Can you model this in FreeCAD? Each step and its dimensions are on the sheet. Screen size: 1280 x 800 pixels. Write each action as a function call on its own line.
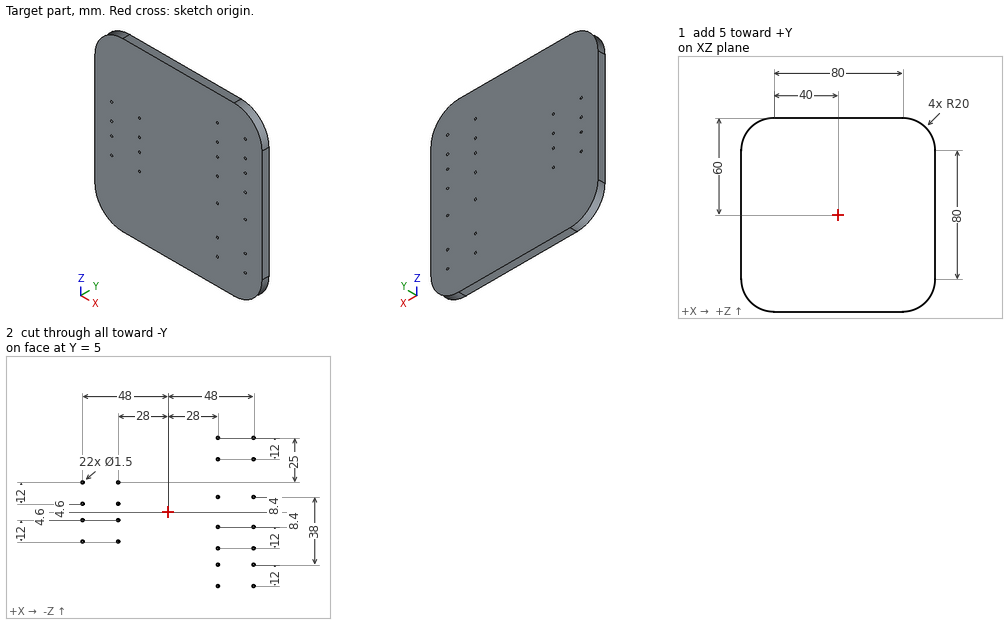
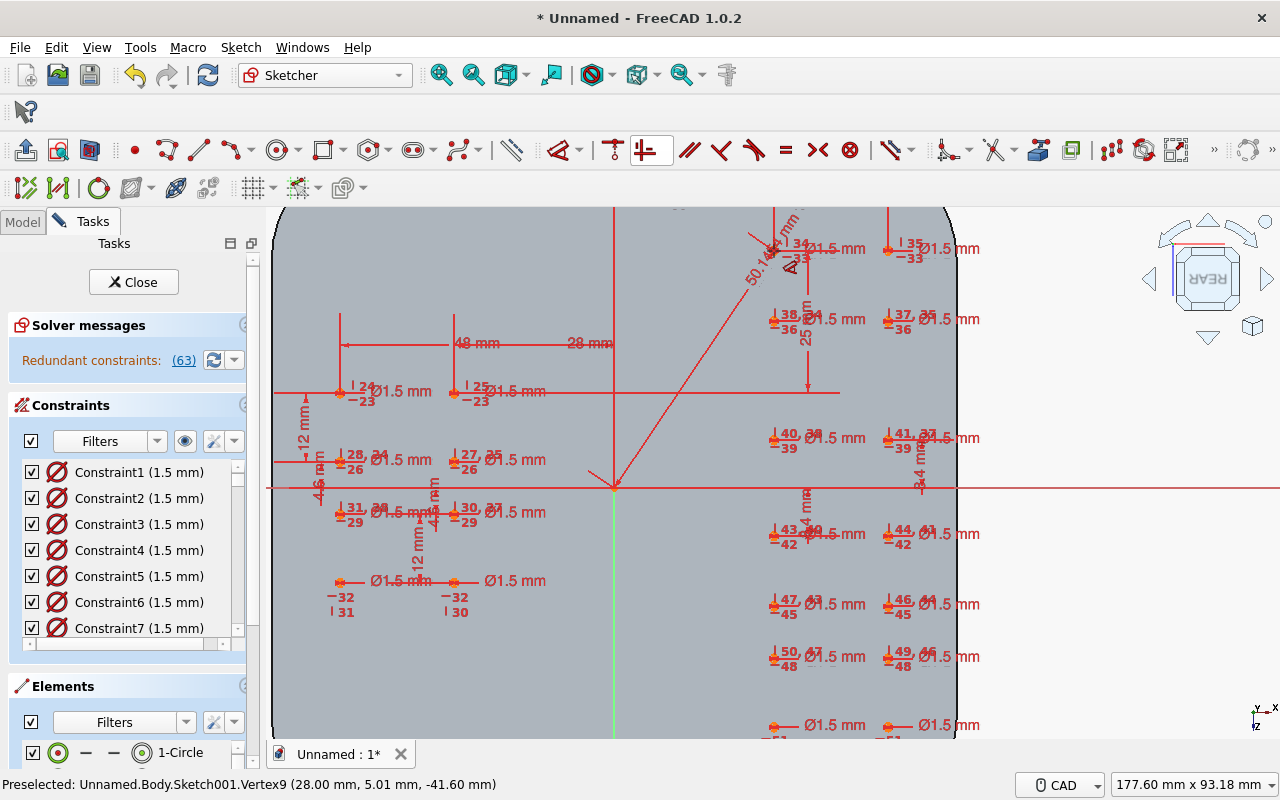
click(774, 321)
click(808, 286)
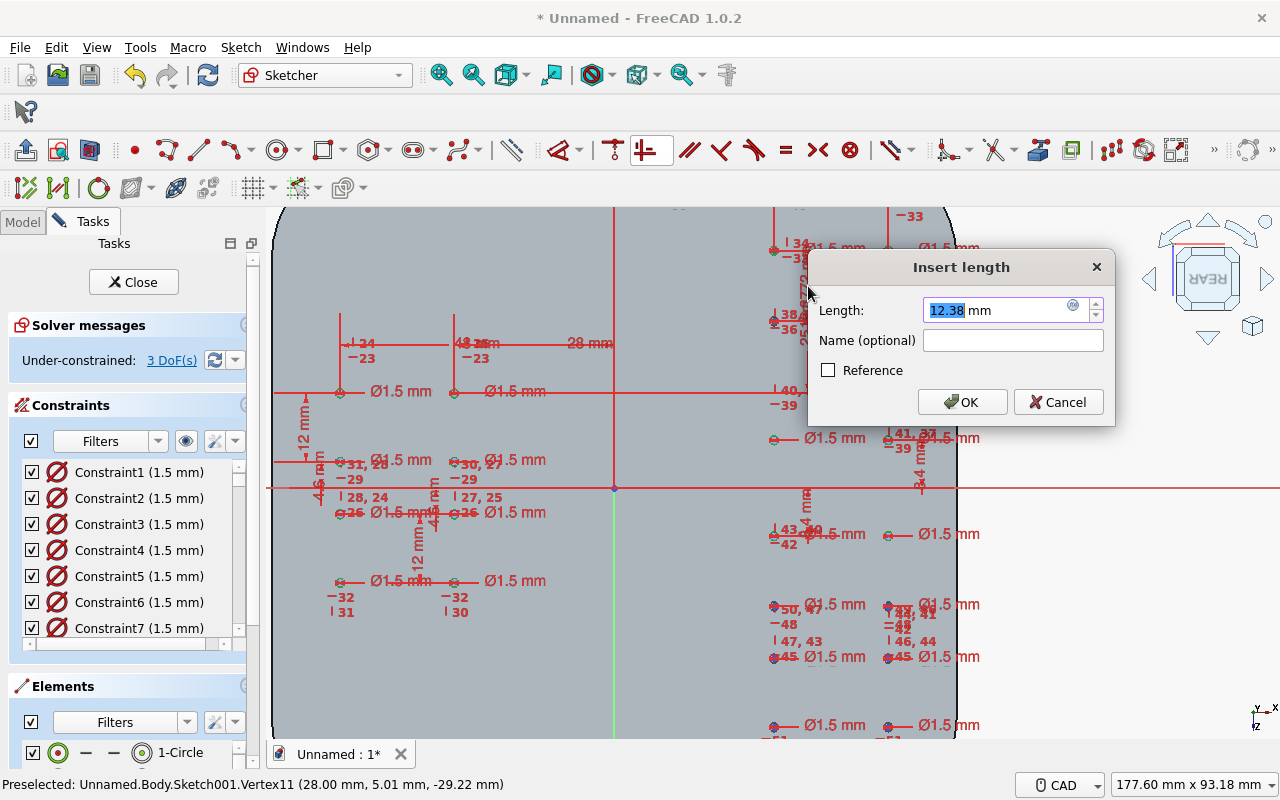
text(12)
key(Return)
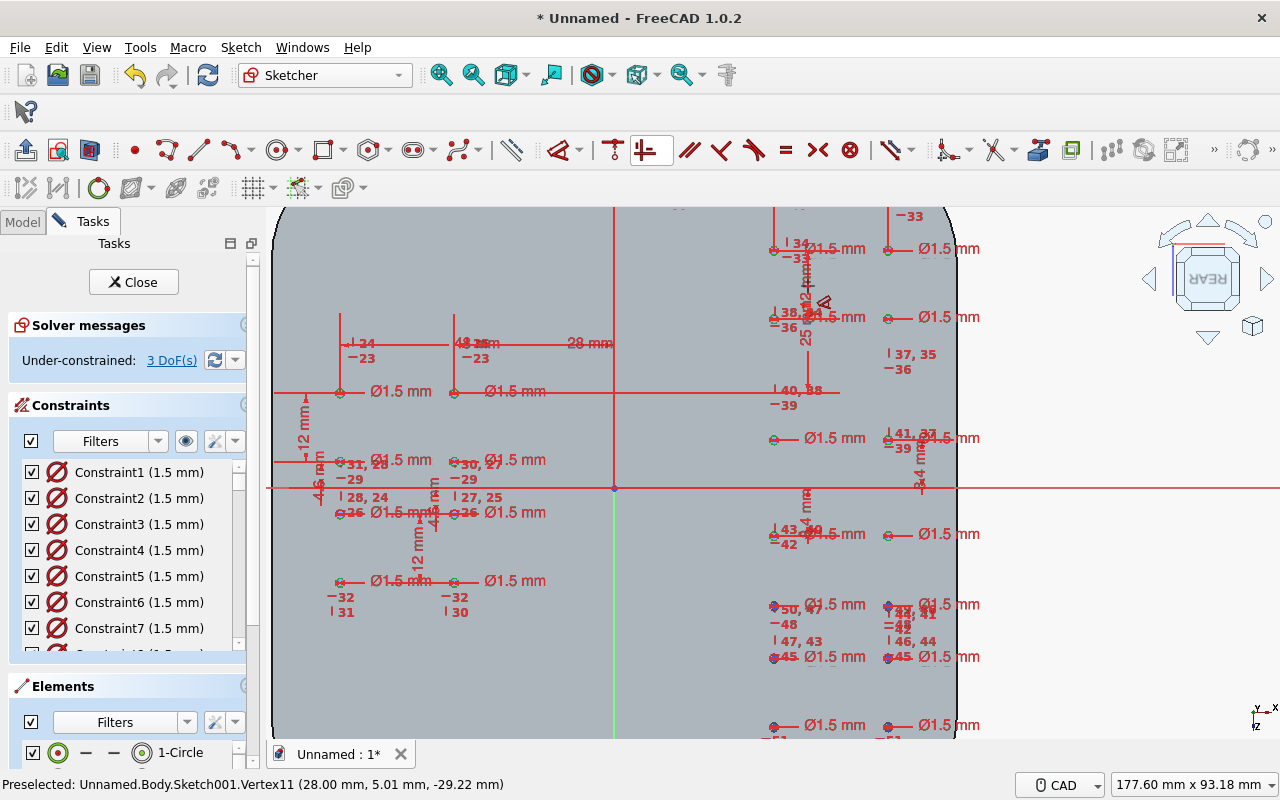
click(774, 536)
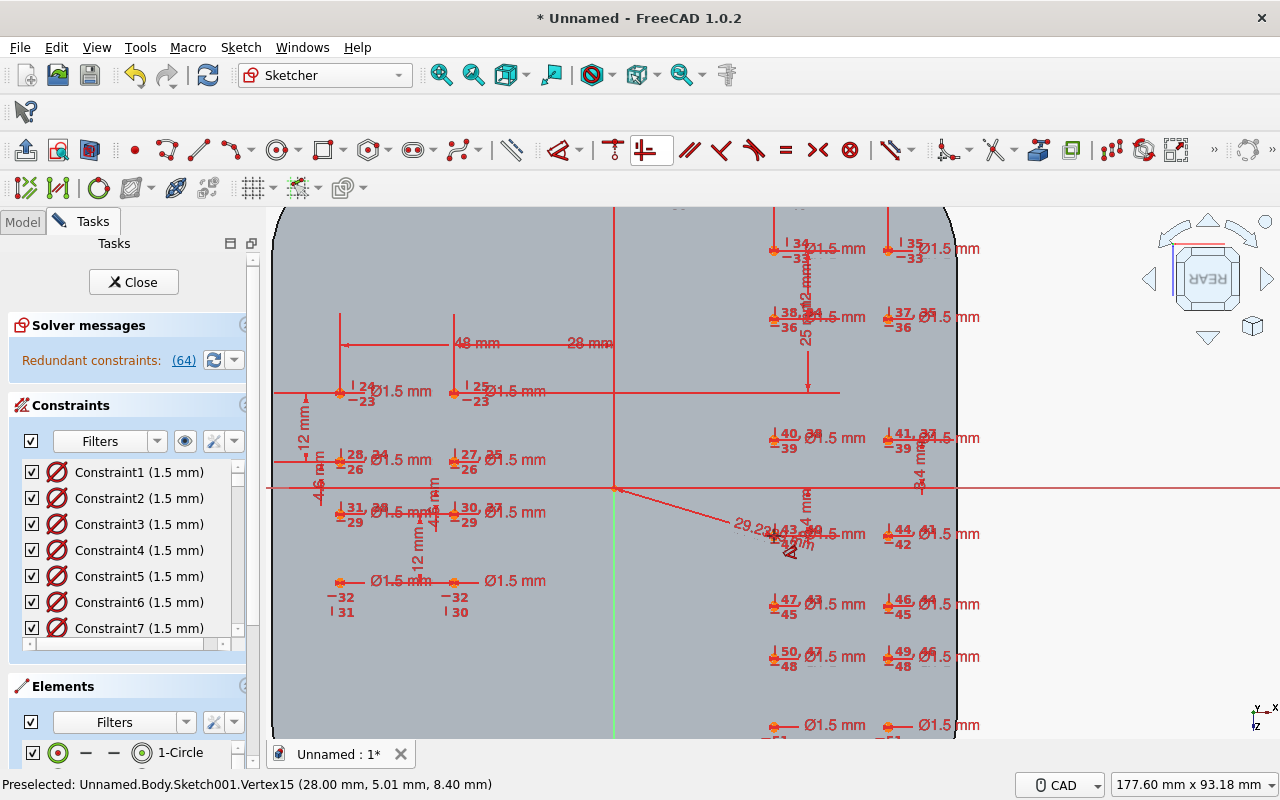
click(774, 606)
click(808, 571)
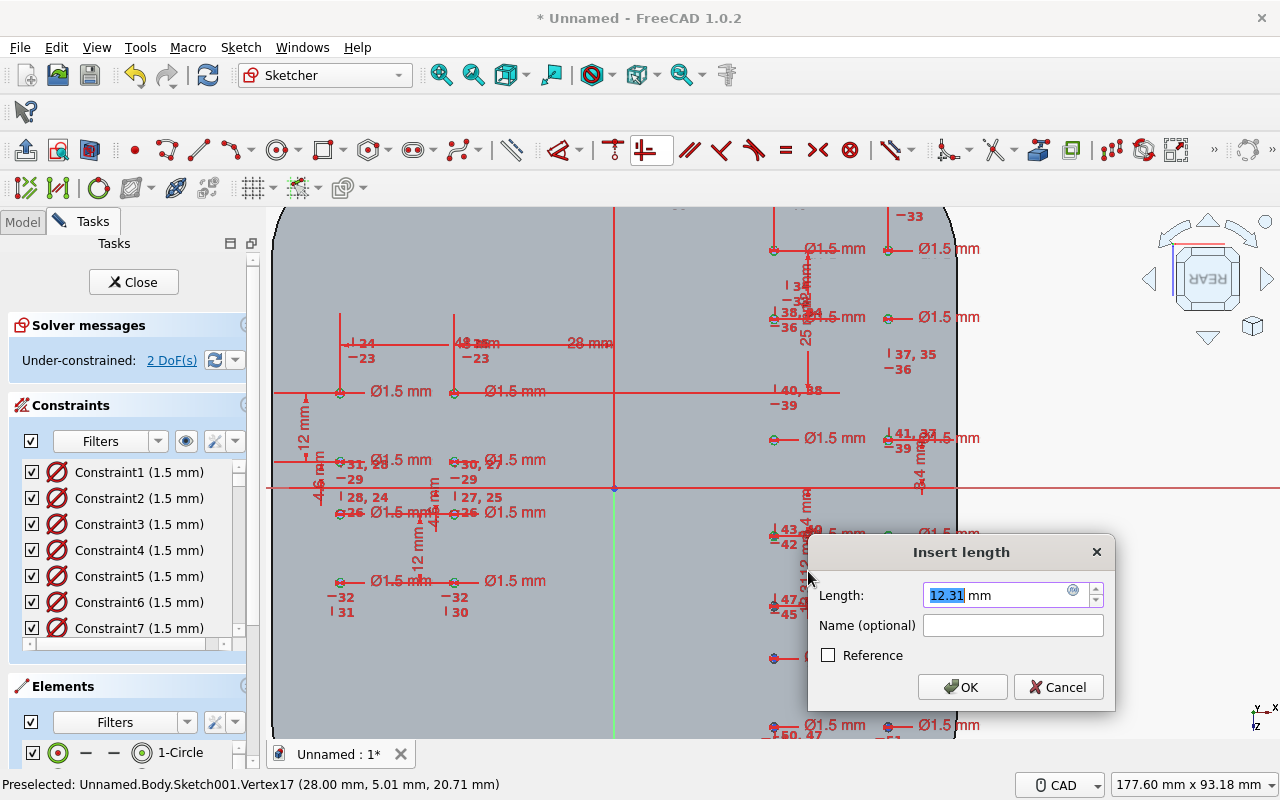
text(12)
key(Return)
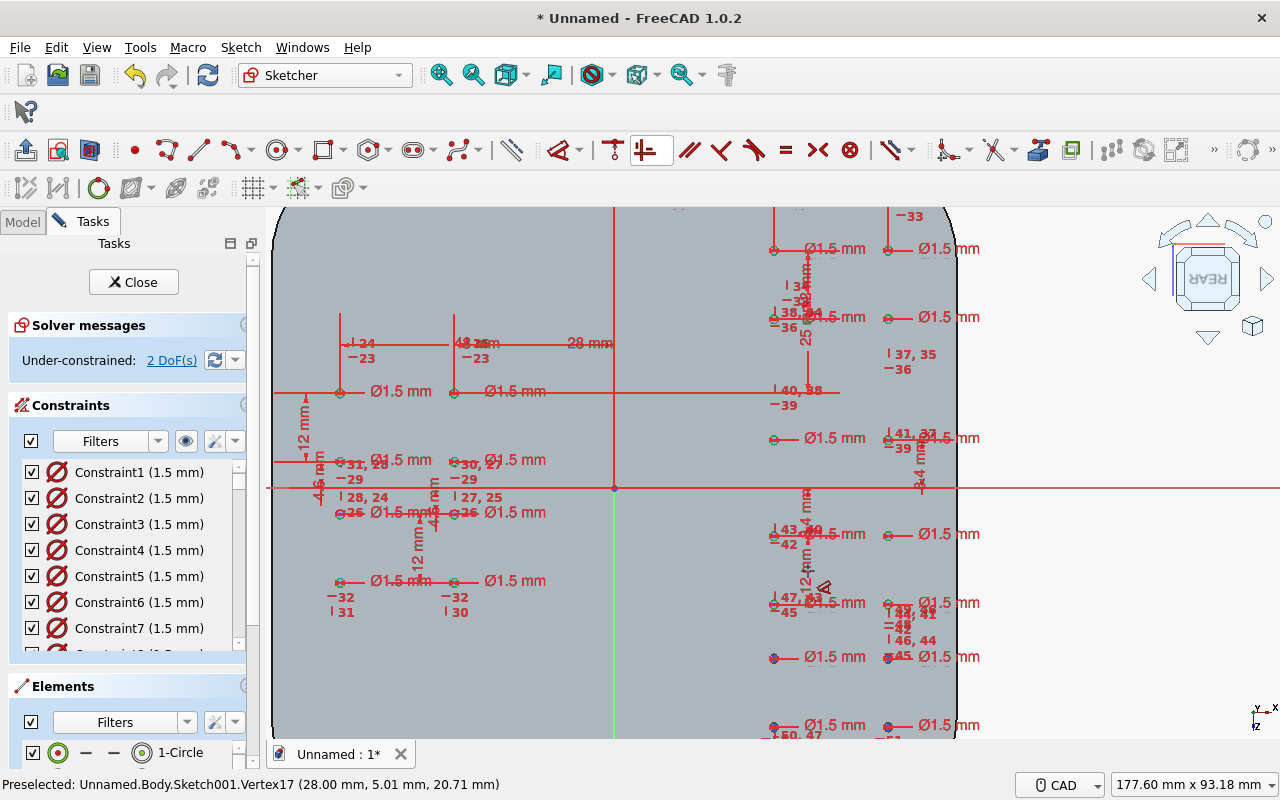
click(888, 440)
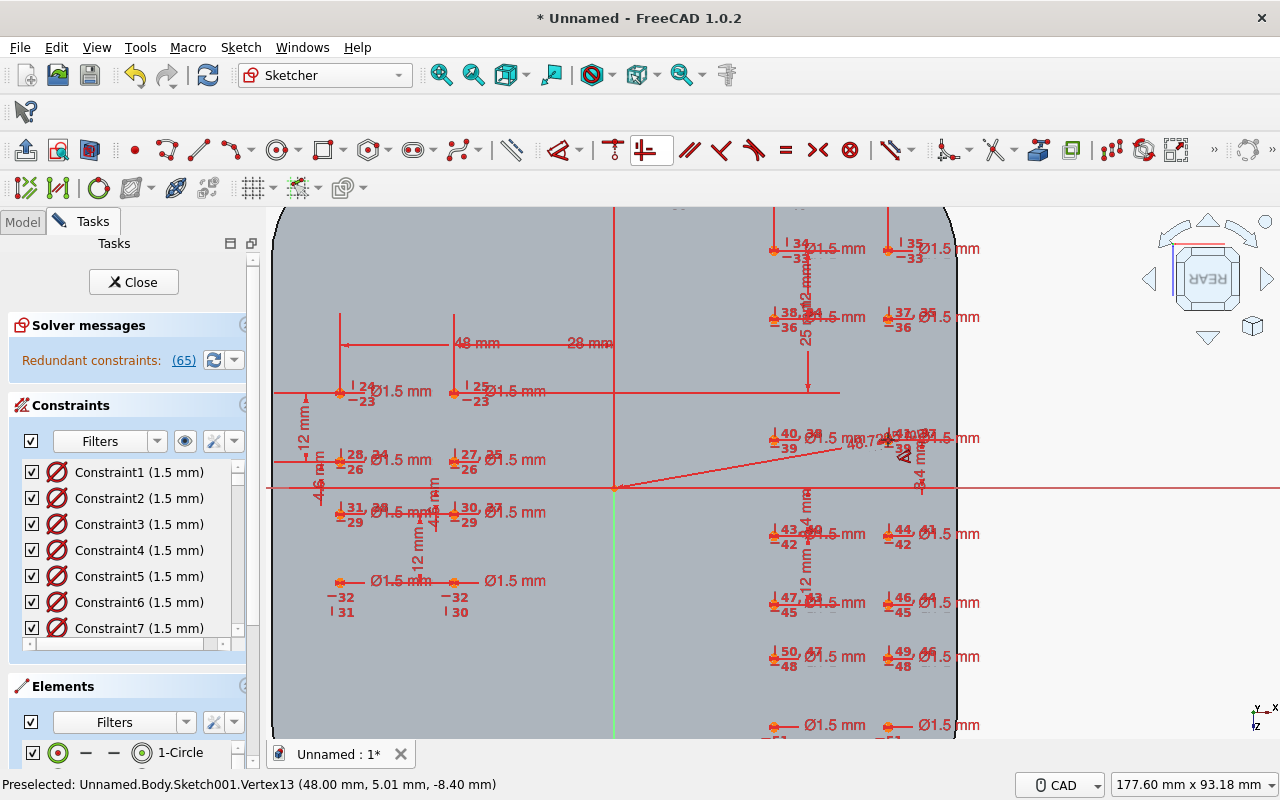
click(888, 659)
click(922, 549)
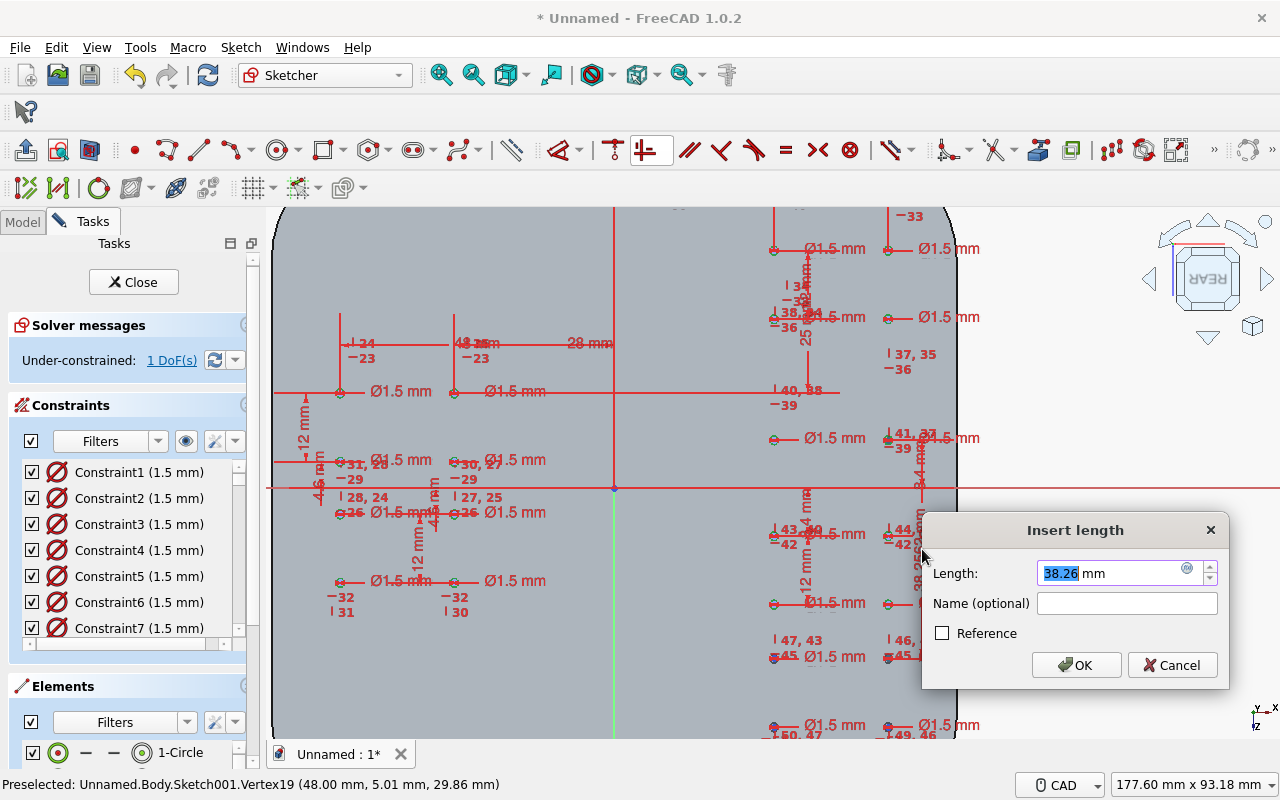
text(38)
key(Return)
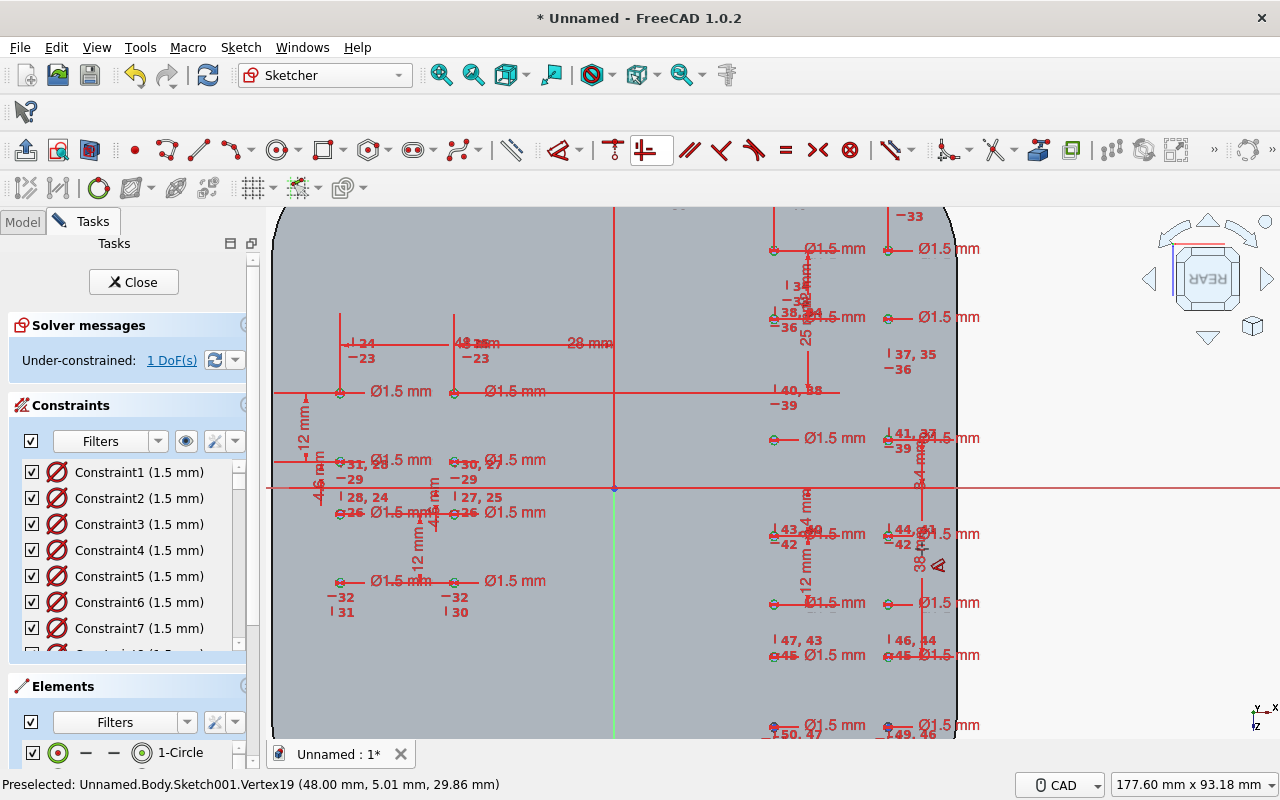
click(888, 657)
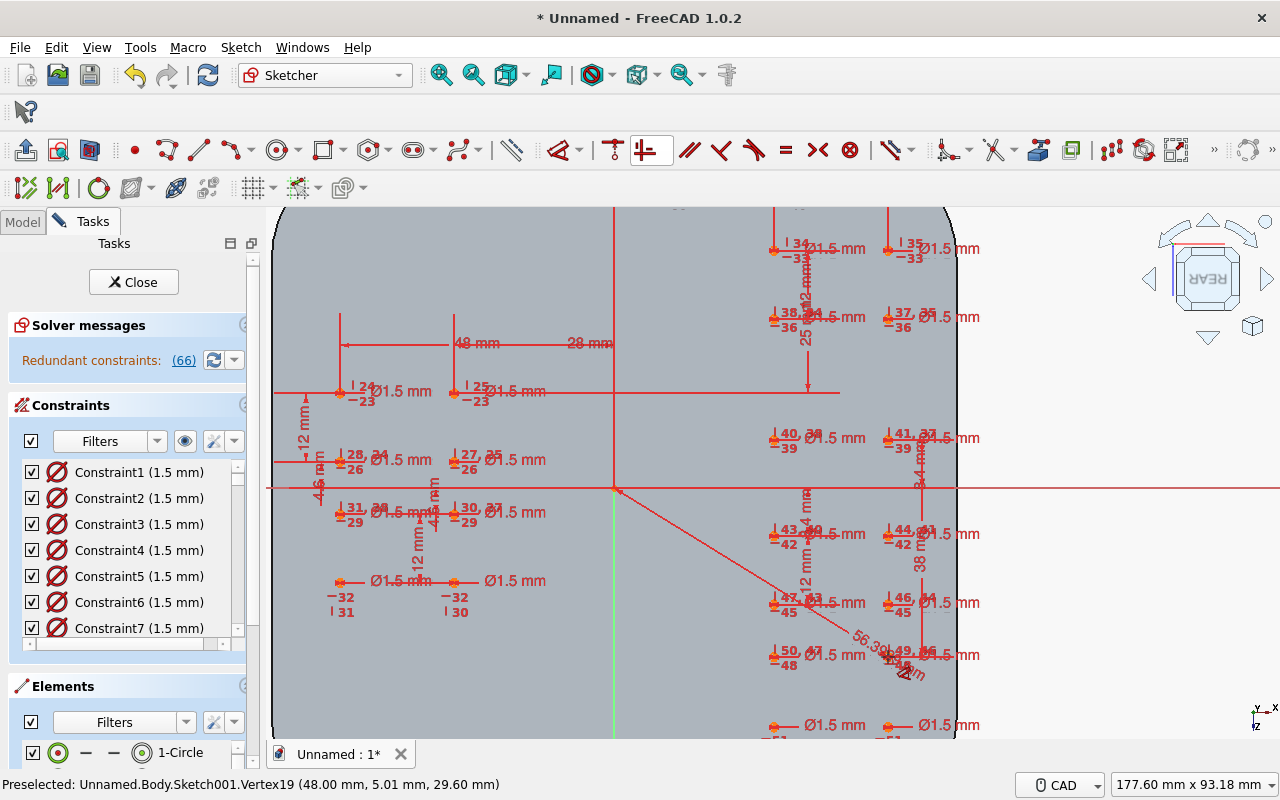
scroll(888, 442, down, 2)